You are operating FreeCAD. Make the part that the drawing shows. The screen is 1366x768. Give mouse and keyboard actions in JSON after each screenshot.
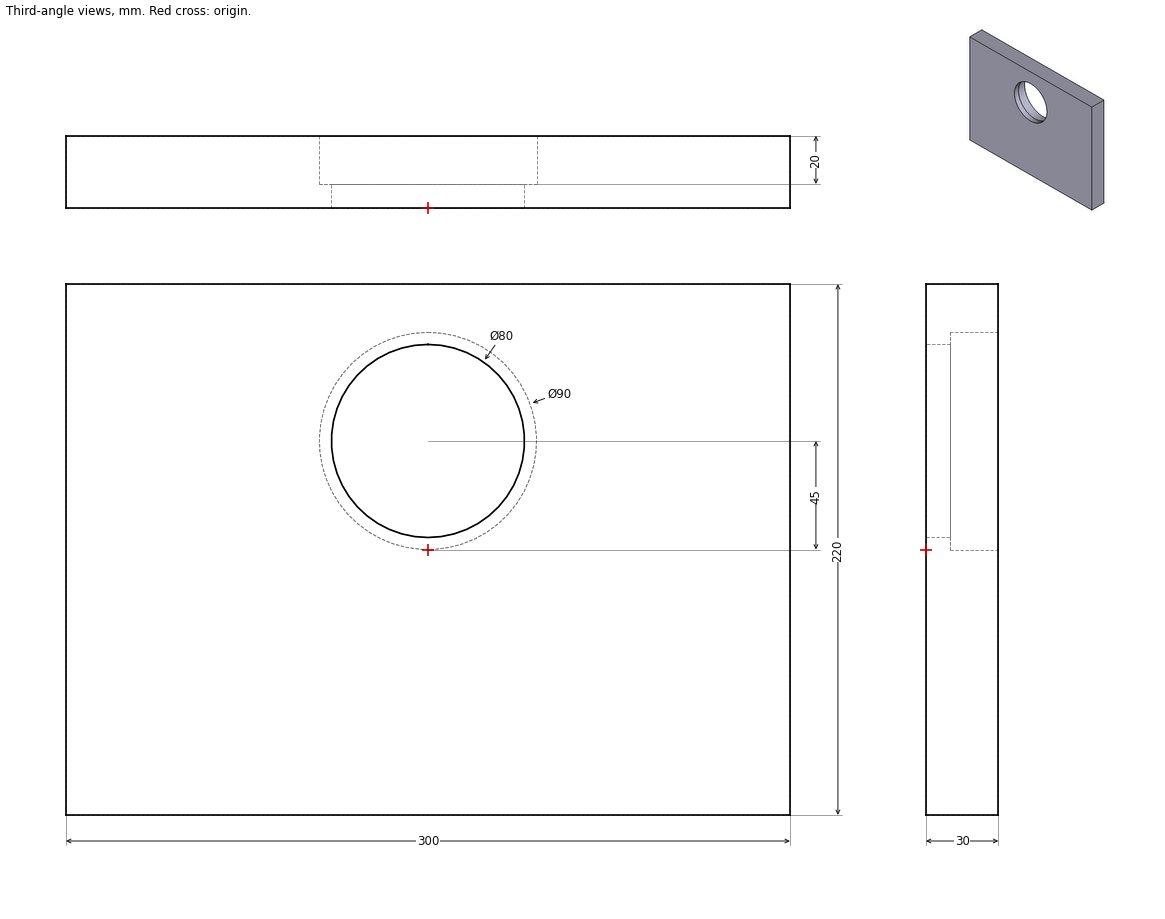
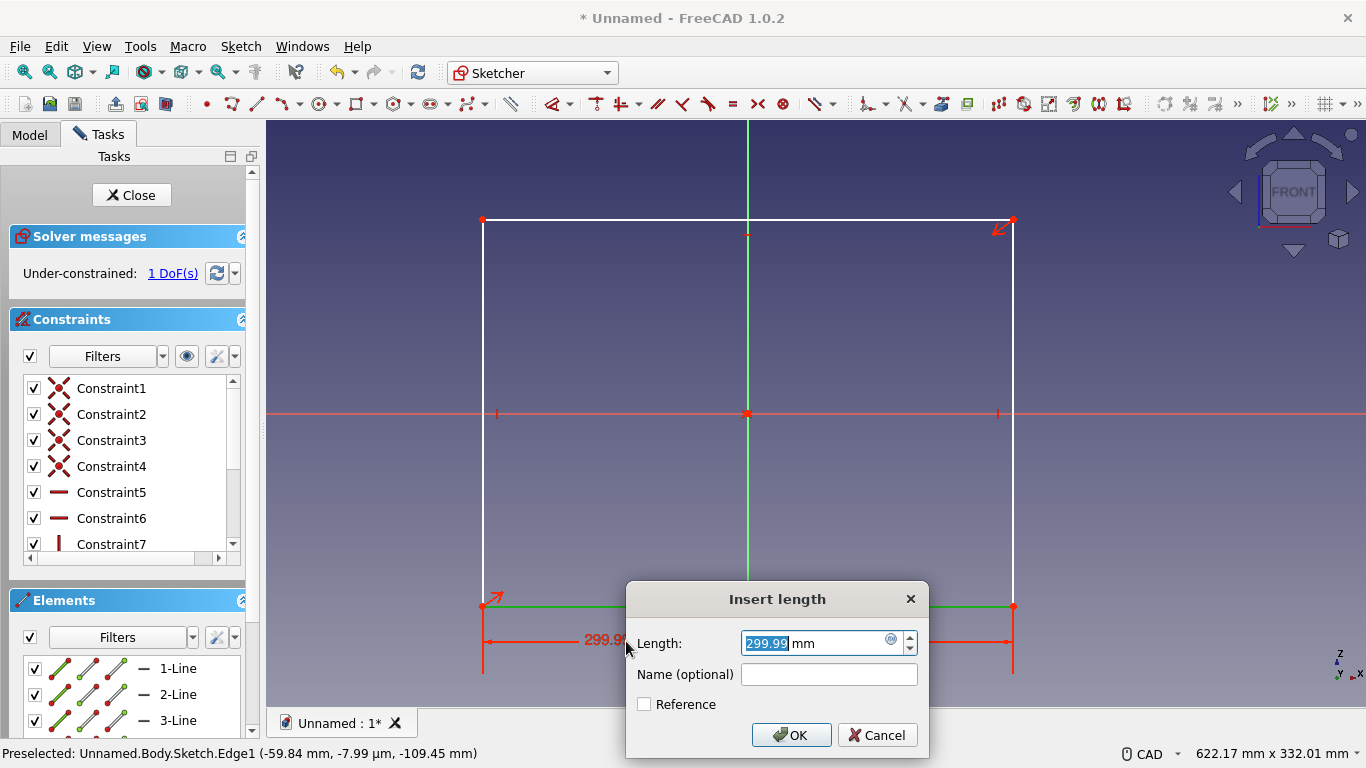
{"action": "type", "text": "300"}
{"action": "key", "text": "Return"}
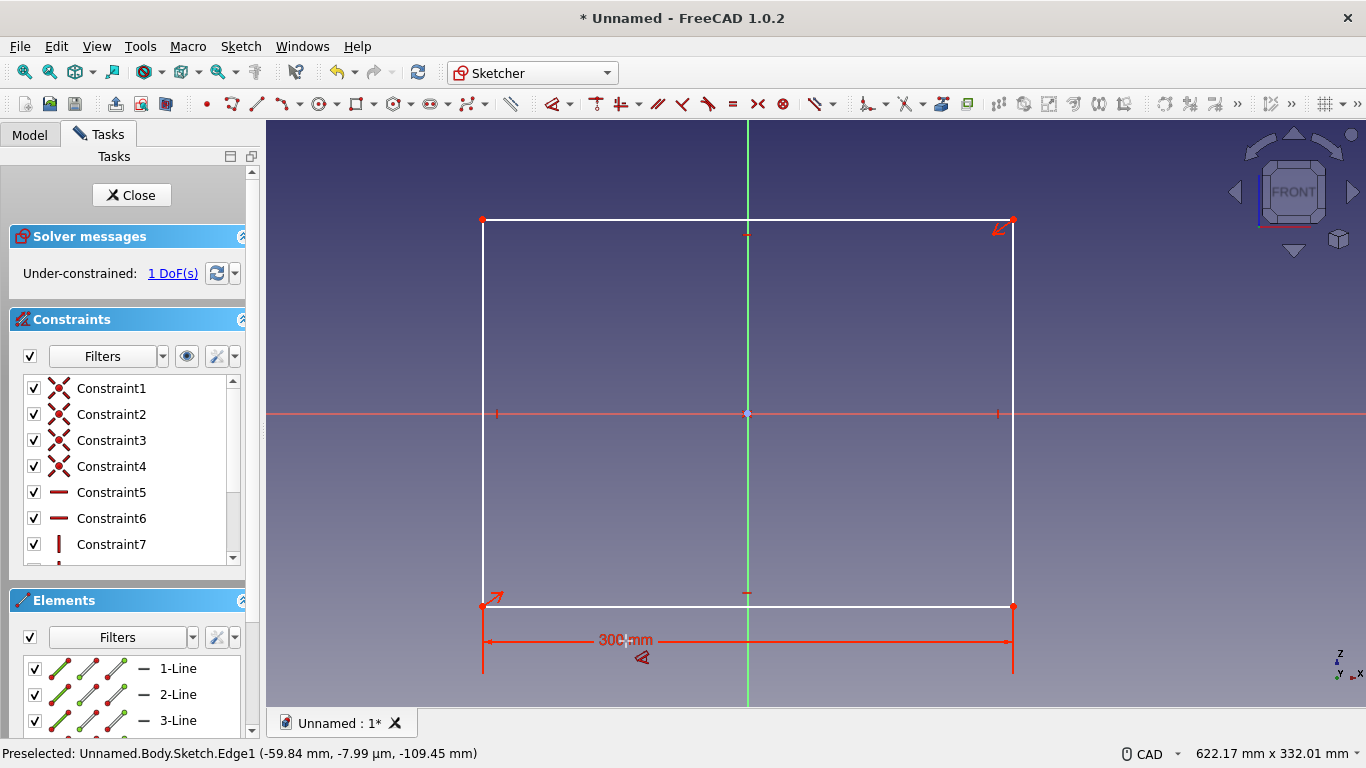
{"action": "left_click", "coordinate": [1013, 491]}
{"action": "left_click", "coordinate": [1047, 324]}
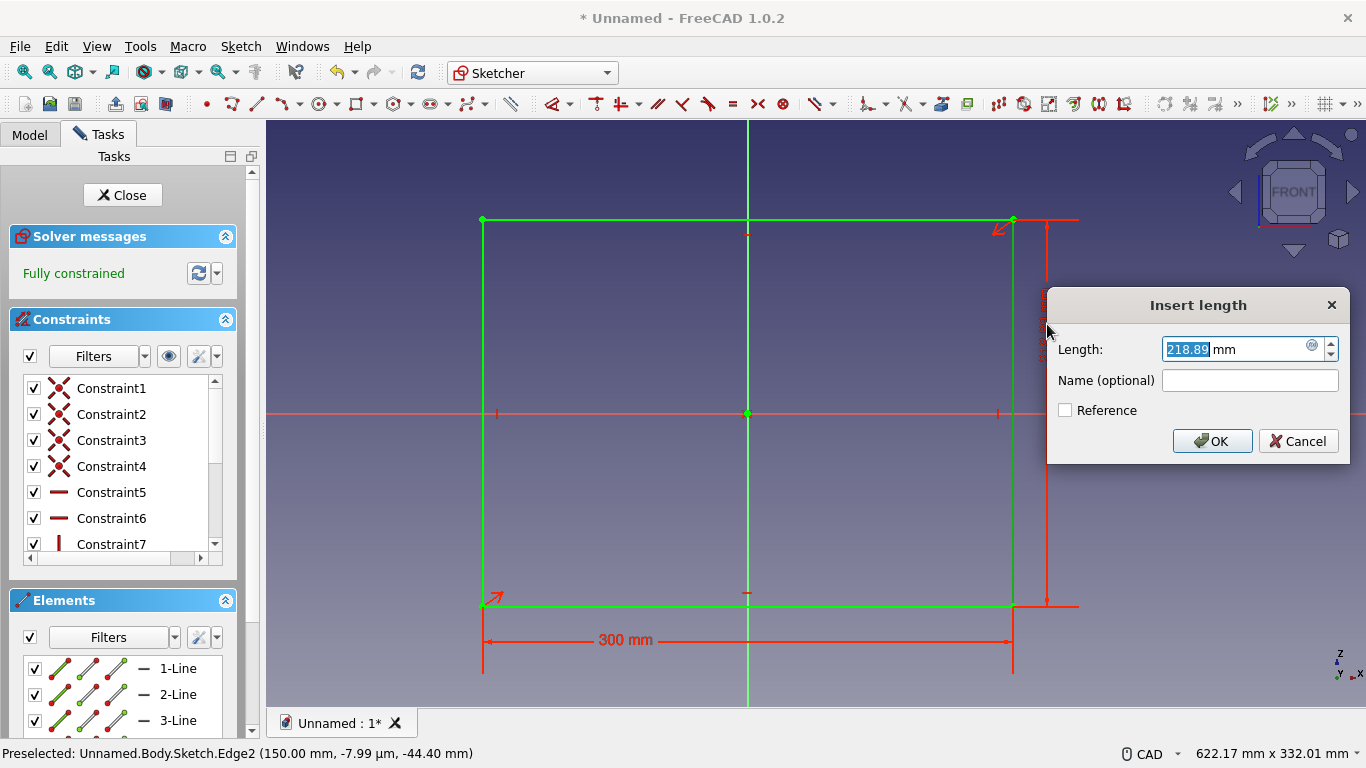
{"action": "type", "text": "220"}
{"action": "key", "text": "Return"}
{"action": "key", "text": "Escape"}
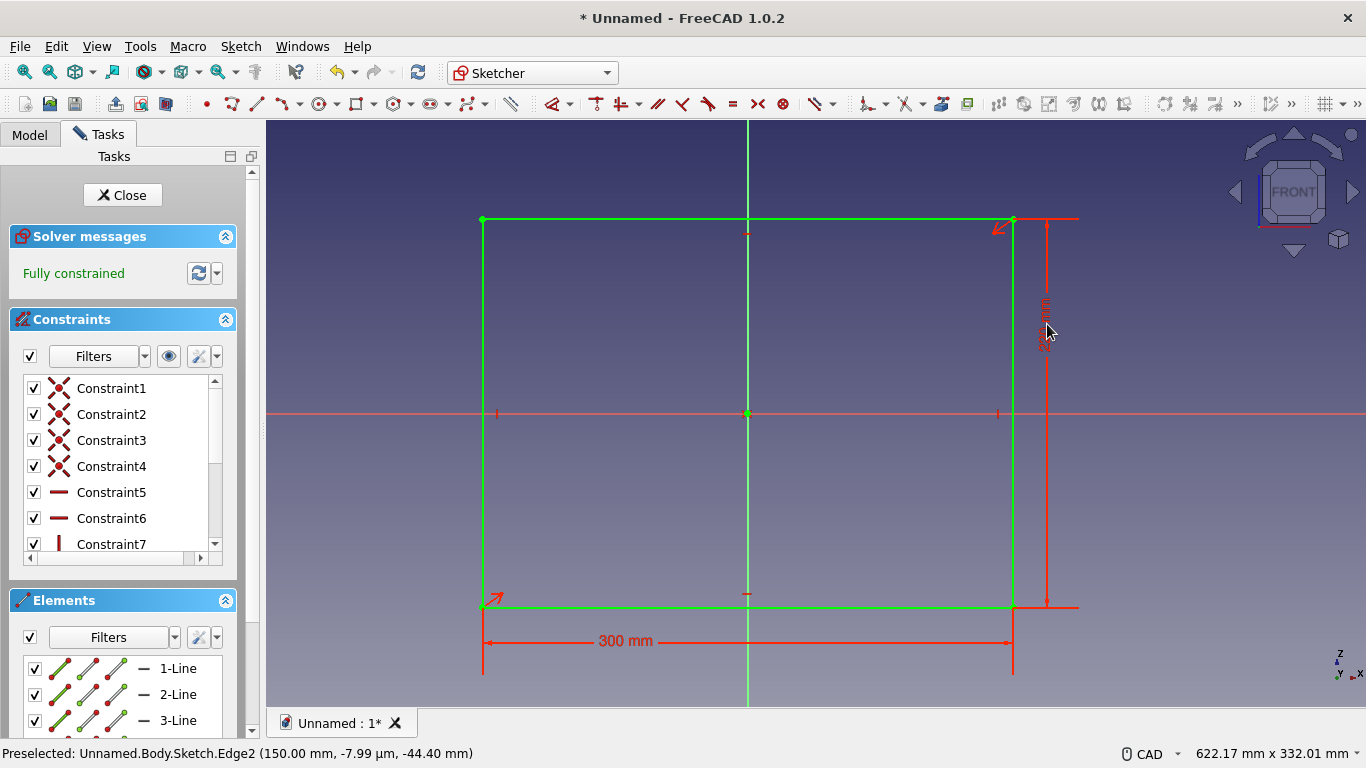
{"action": "left_click", "coordinate": [123, 195]}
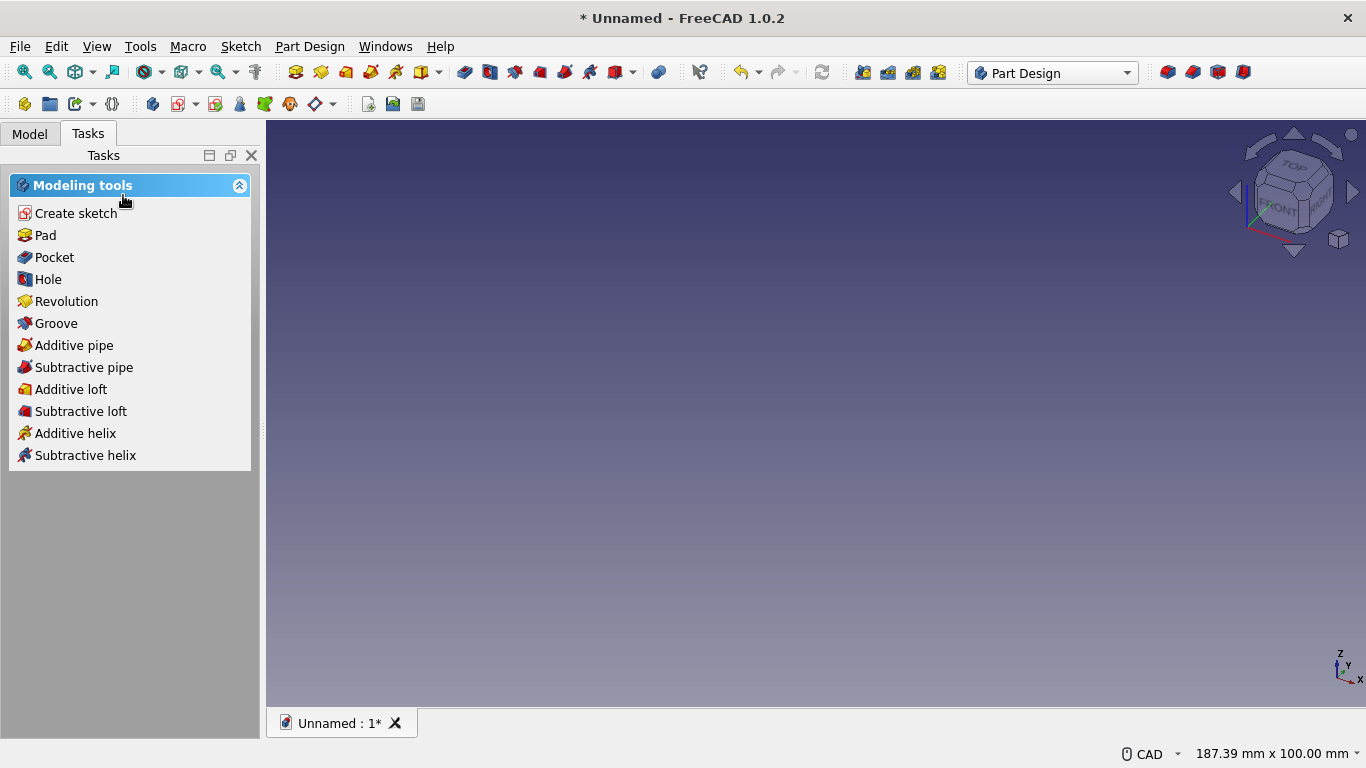
{"action": "left_click", "coordinate": [296, 72]}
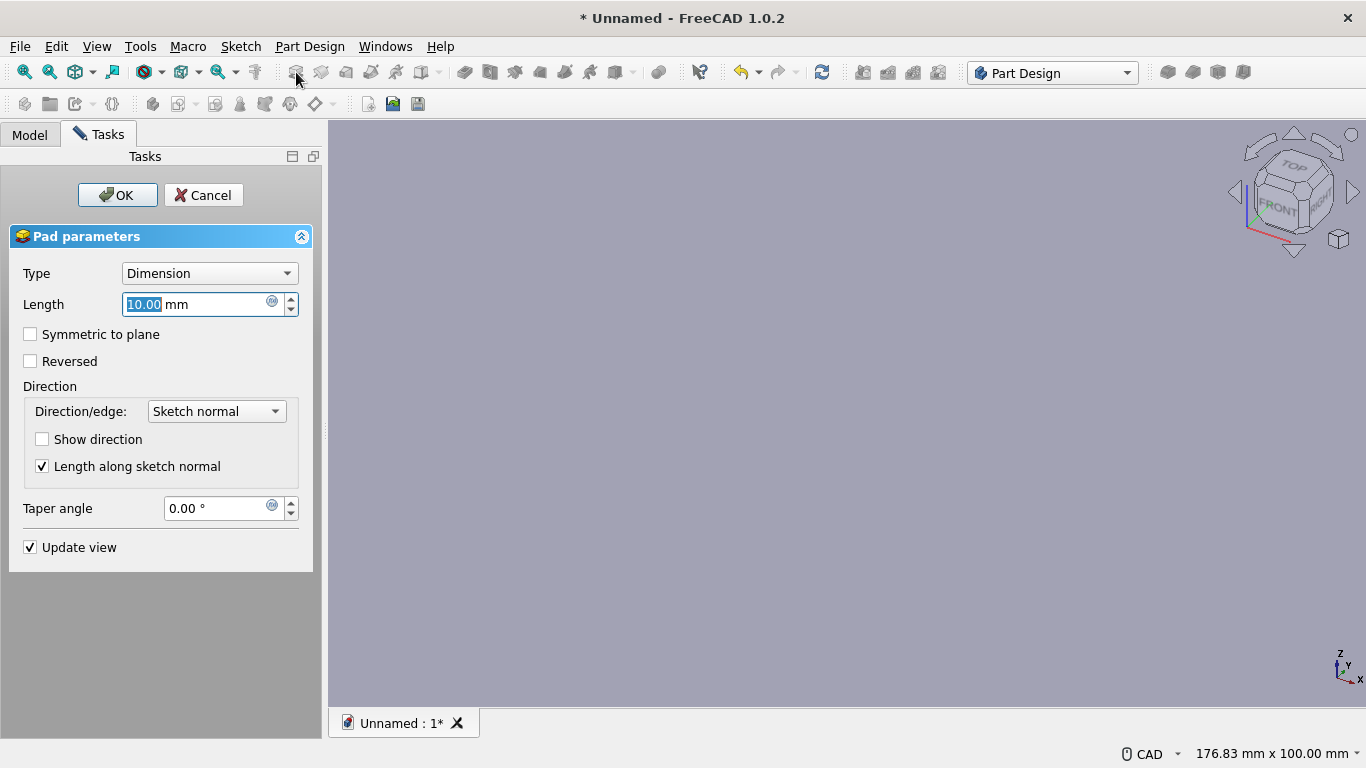
{"action": "type", "text": "30"}
{"action": "key", "text": "Tab"}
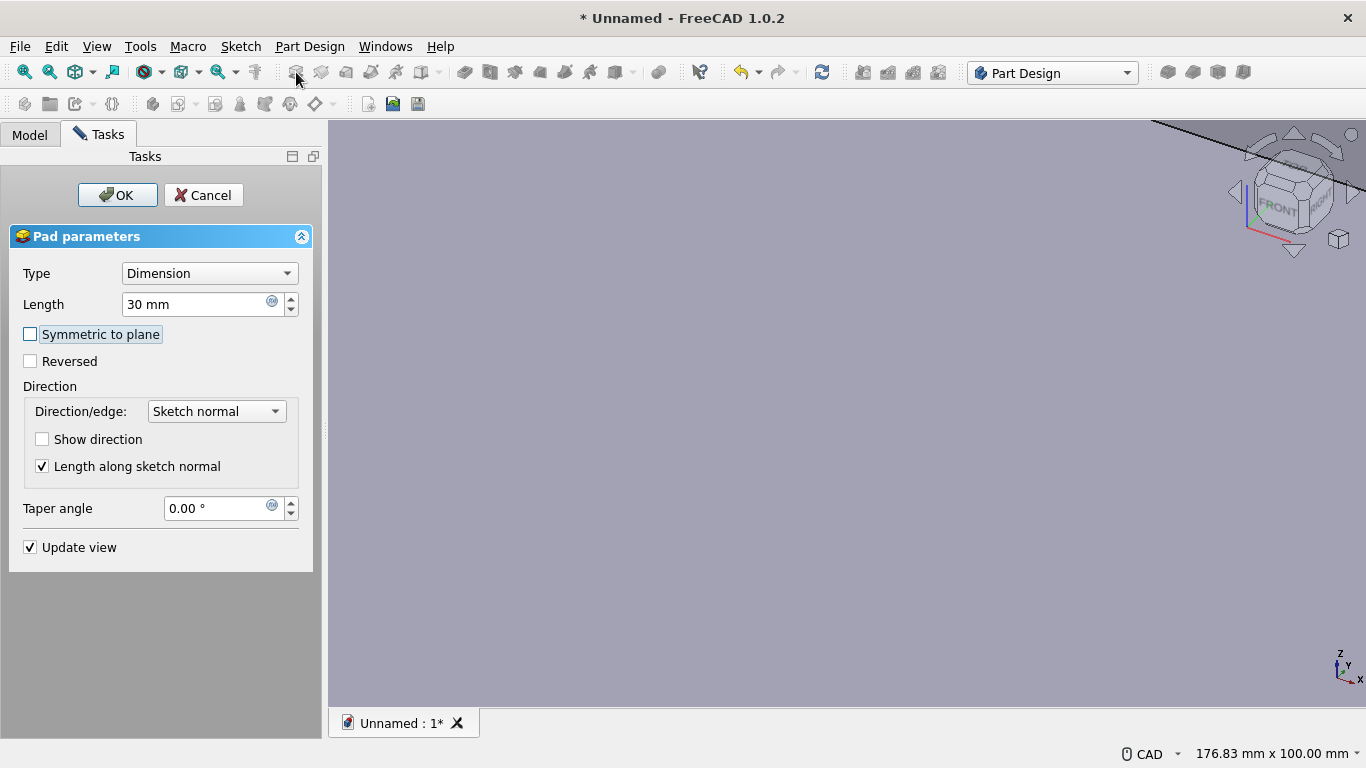
{"action": "left_click", "coordinate": [31, 361]}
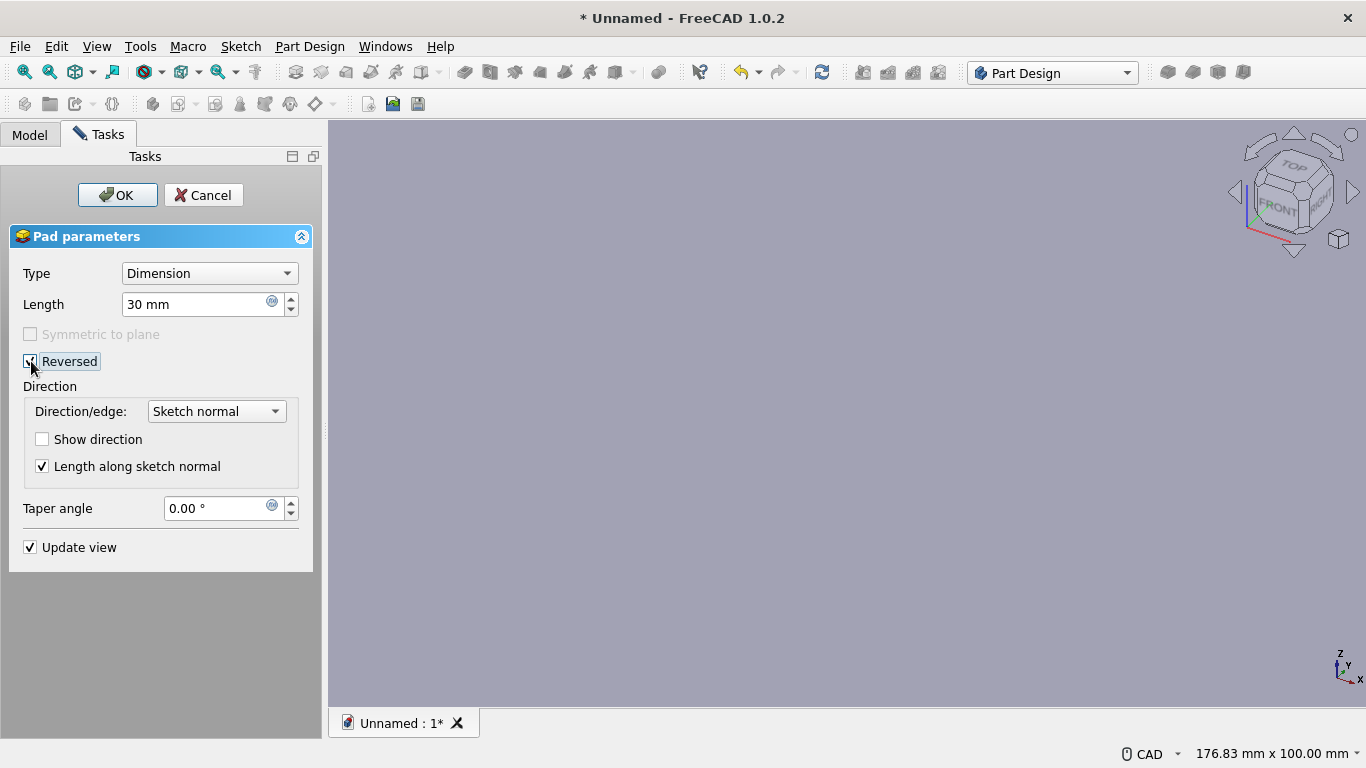
{"action": "left_click", "coordinate": [118, 195]}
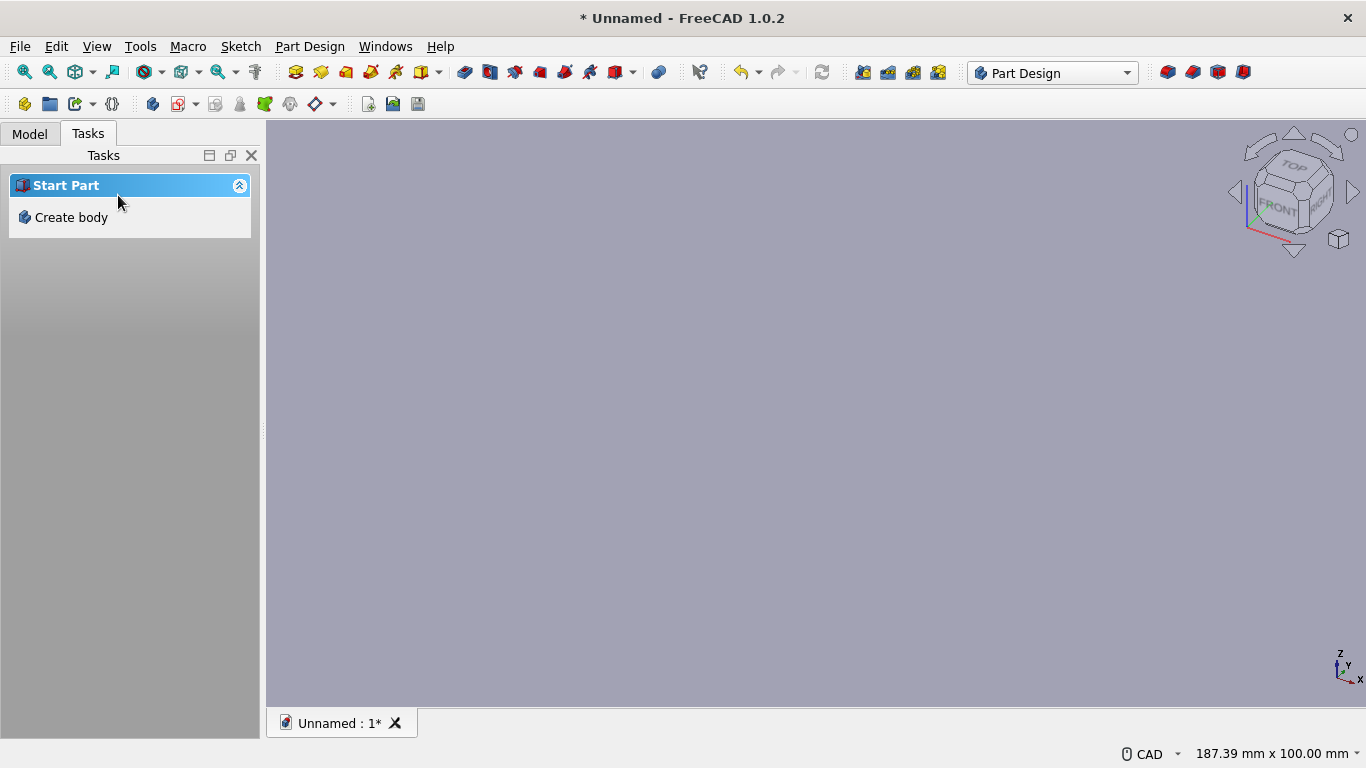
{"action": "key", "text": "v f"}